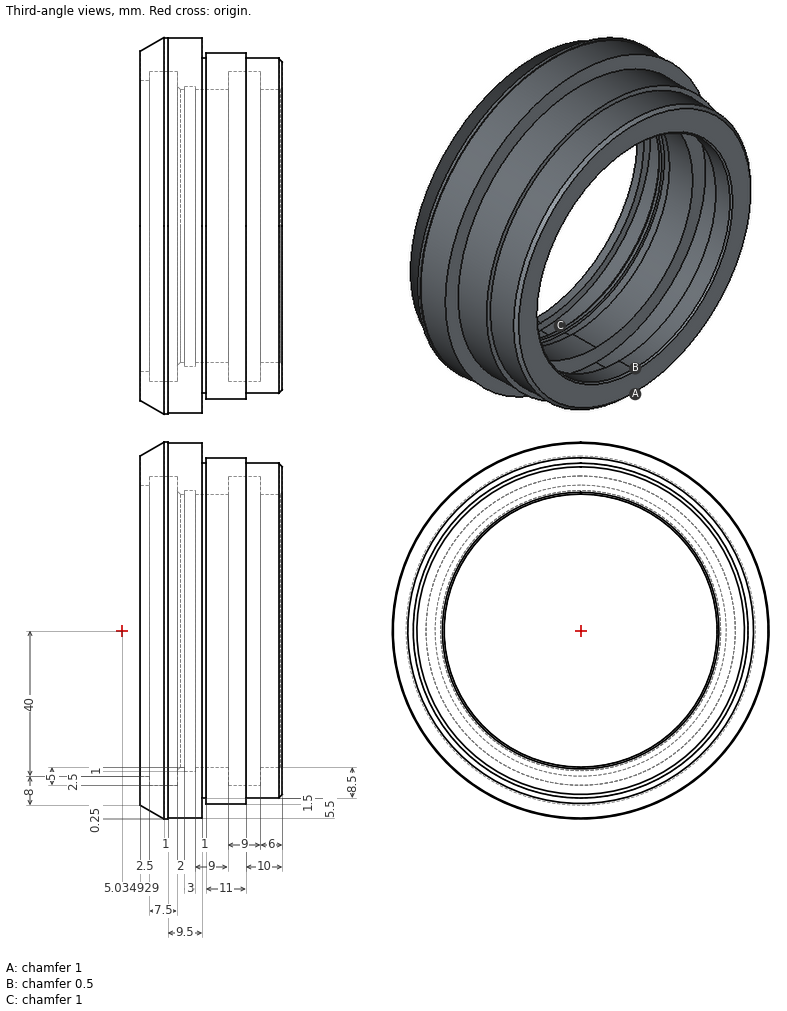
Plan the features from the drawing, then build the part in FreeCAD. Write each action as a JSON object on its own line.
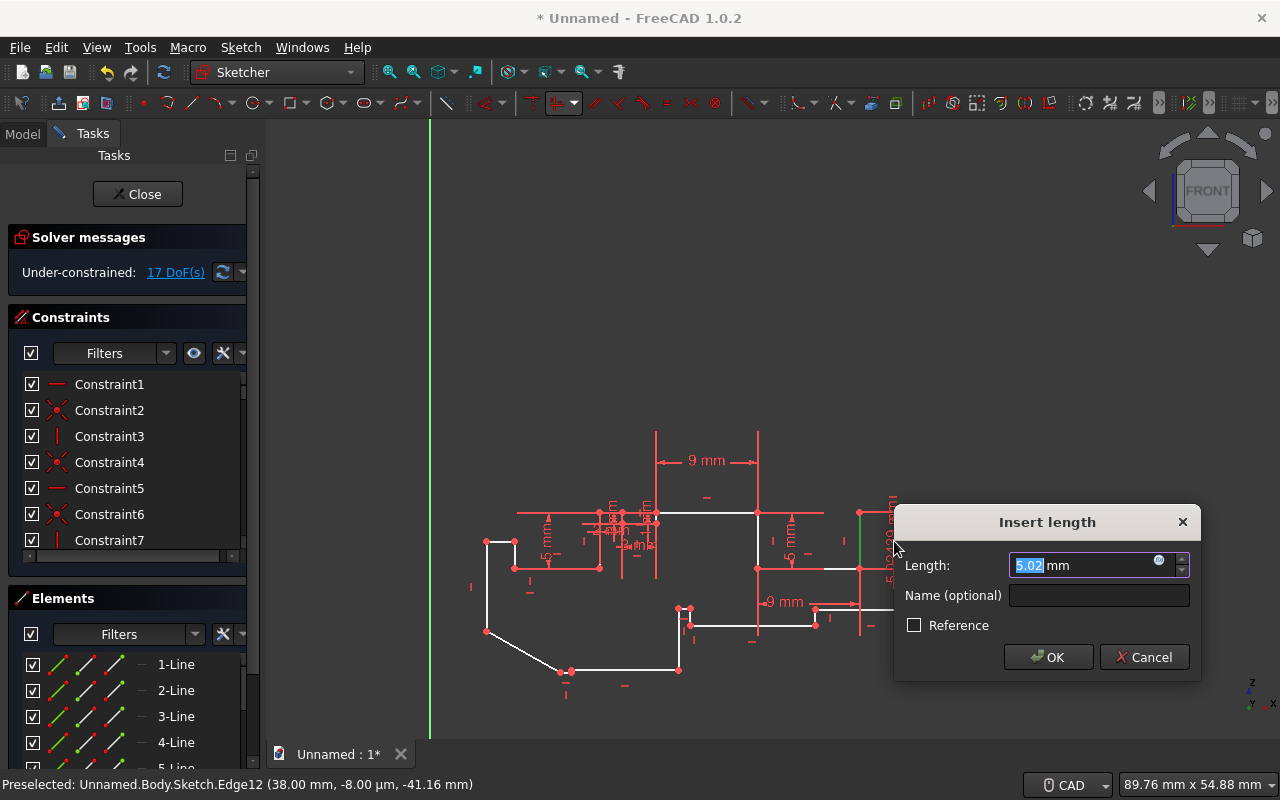
{"action": "type", "text": "5"}
{"action": "key", "text": "Return"}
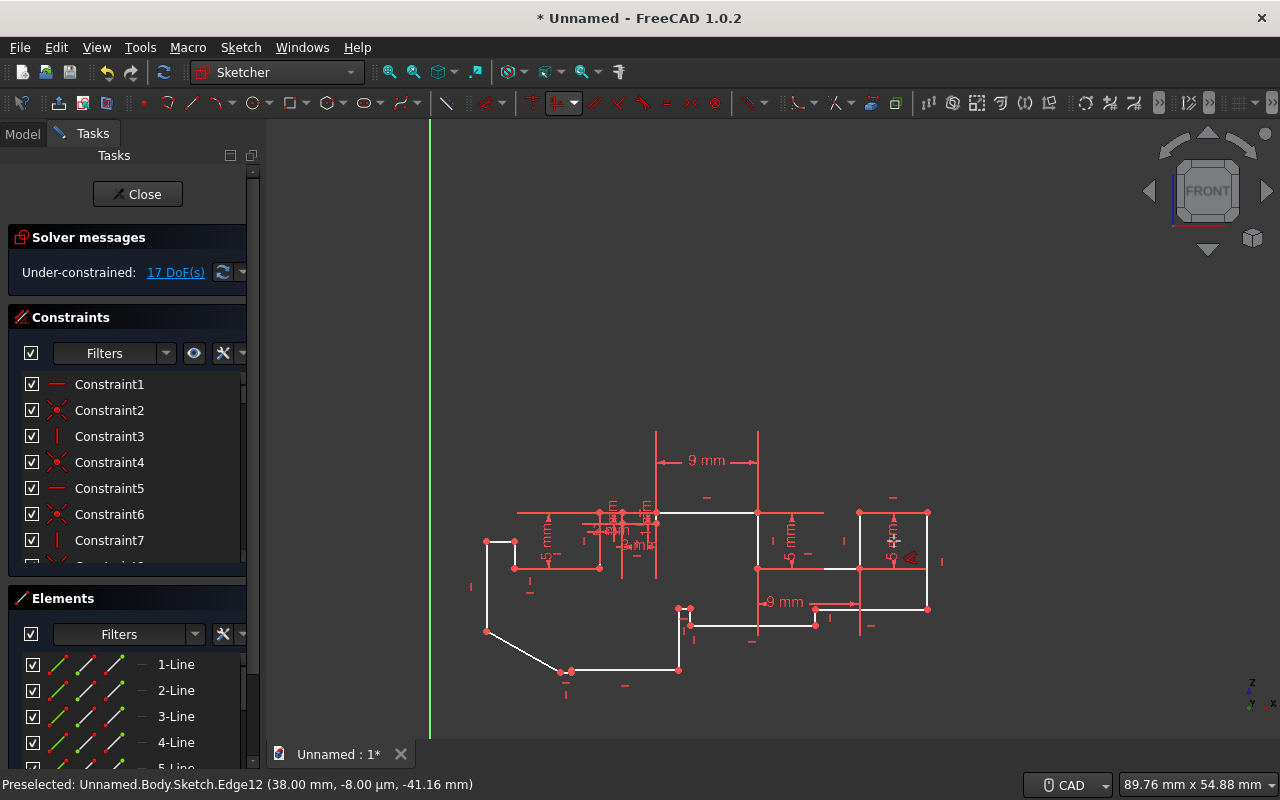
{"action": "left_click", "coordinate": [880, 513]}
{"action": "left_click", "coordinate": [893, 479]}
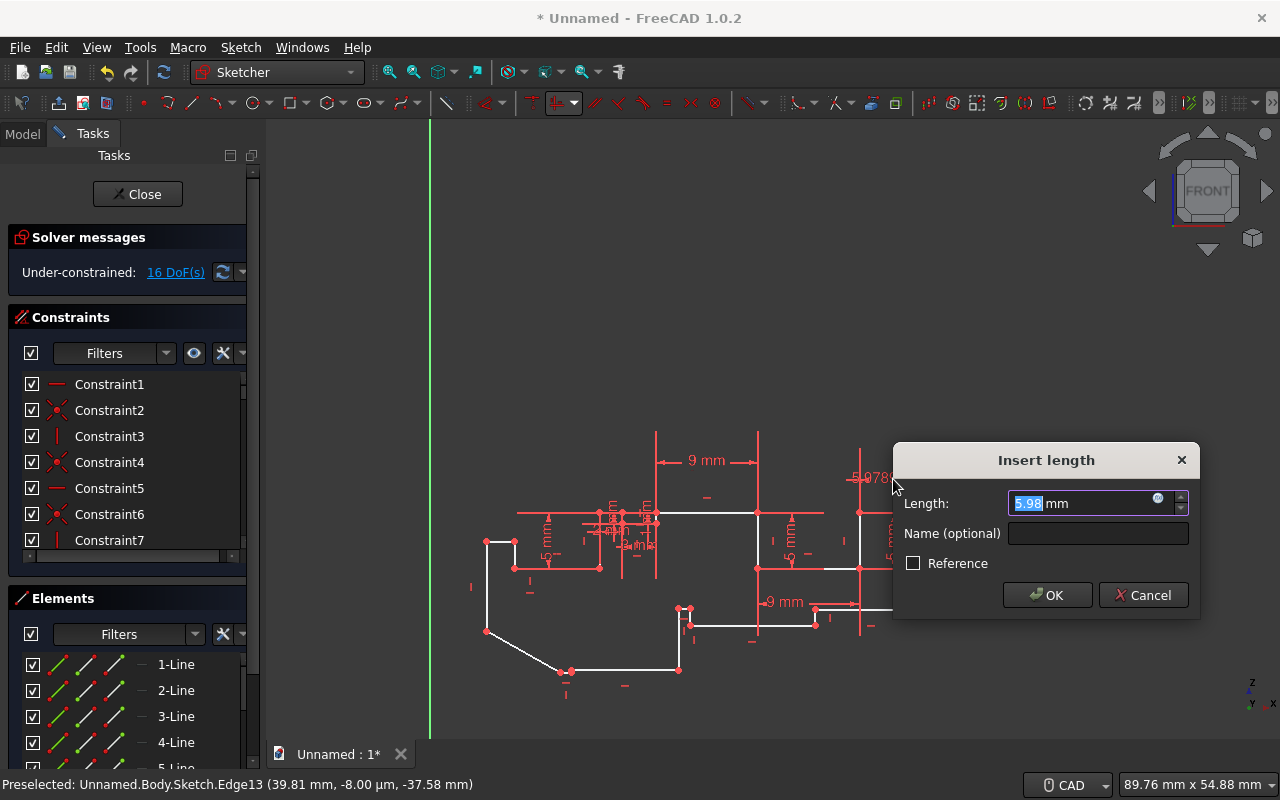
{"action": "type", "text": "6"}
{"action": "key", "text": "Return"}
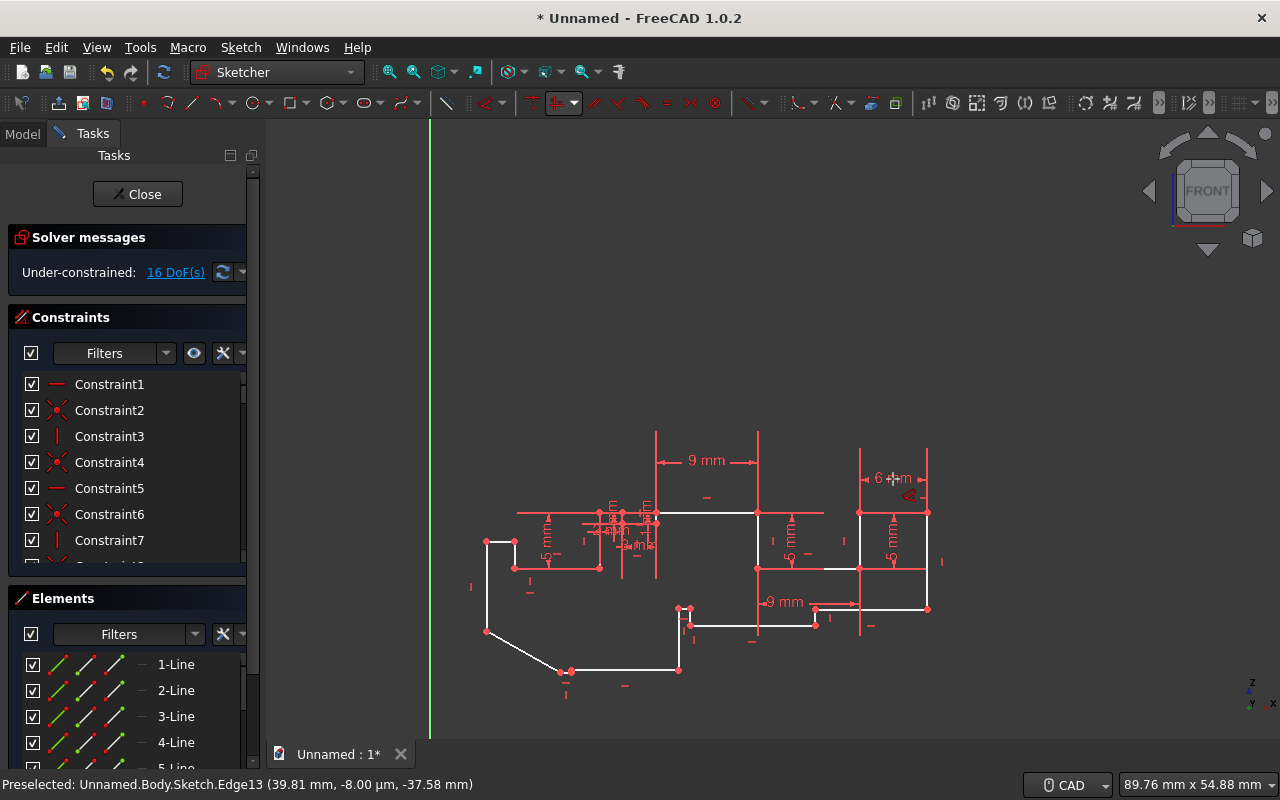
{"action": "scroll", "coordinate": [685, 609], "scroll_direction": "up", "scroll_amount": 7}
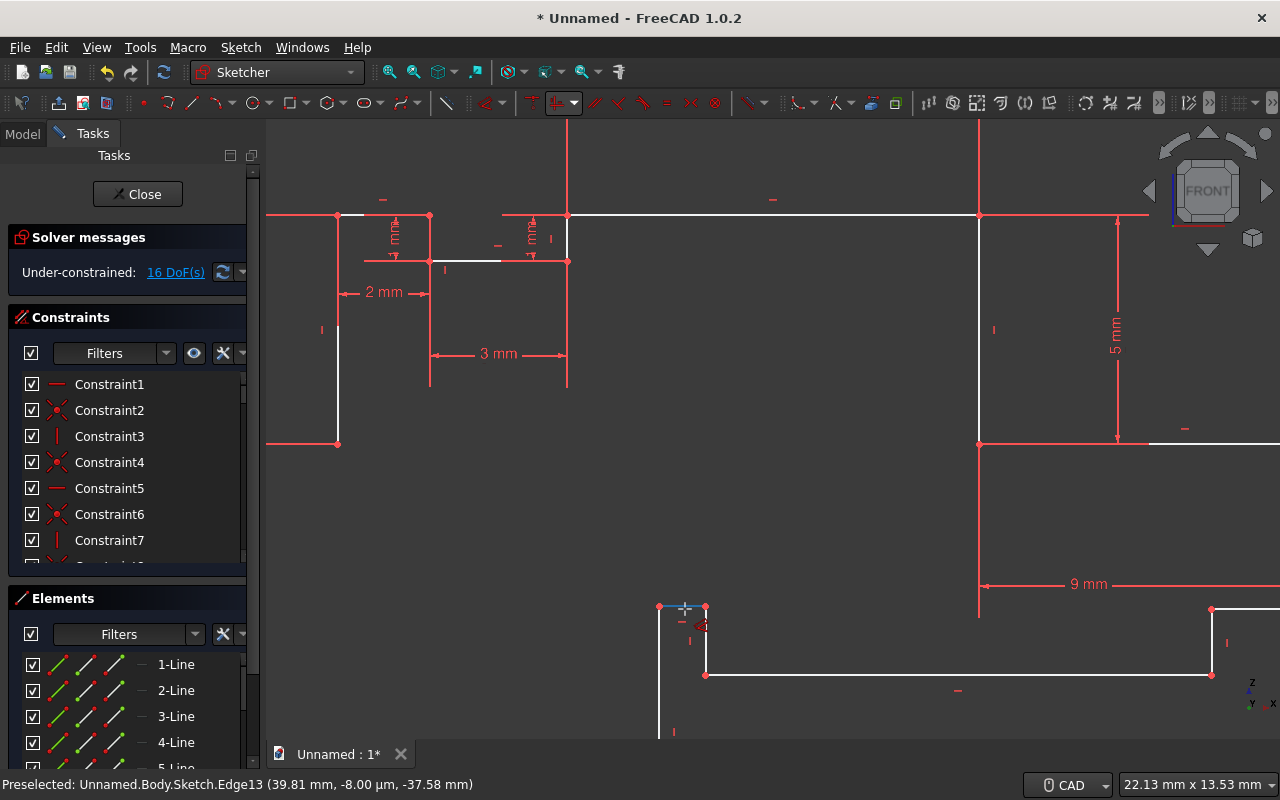
{"action": "left_click", "coordinate": [683, 606]}
{"action": "left_click", "coordinate": [683, 640]}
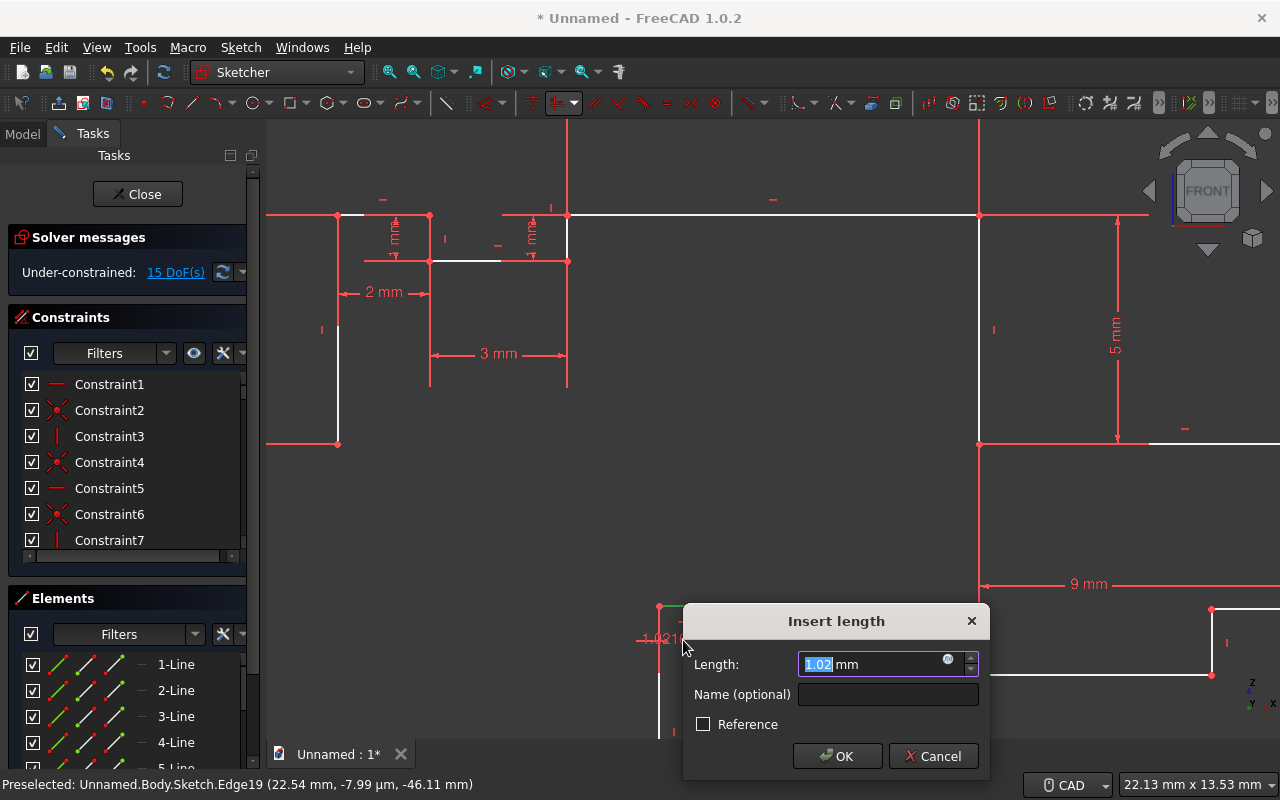
{"action": "type", "text": "1"}
{"action": "key", "text": "Return"}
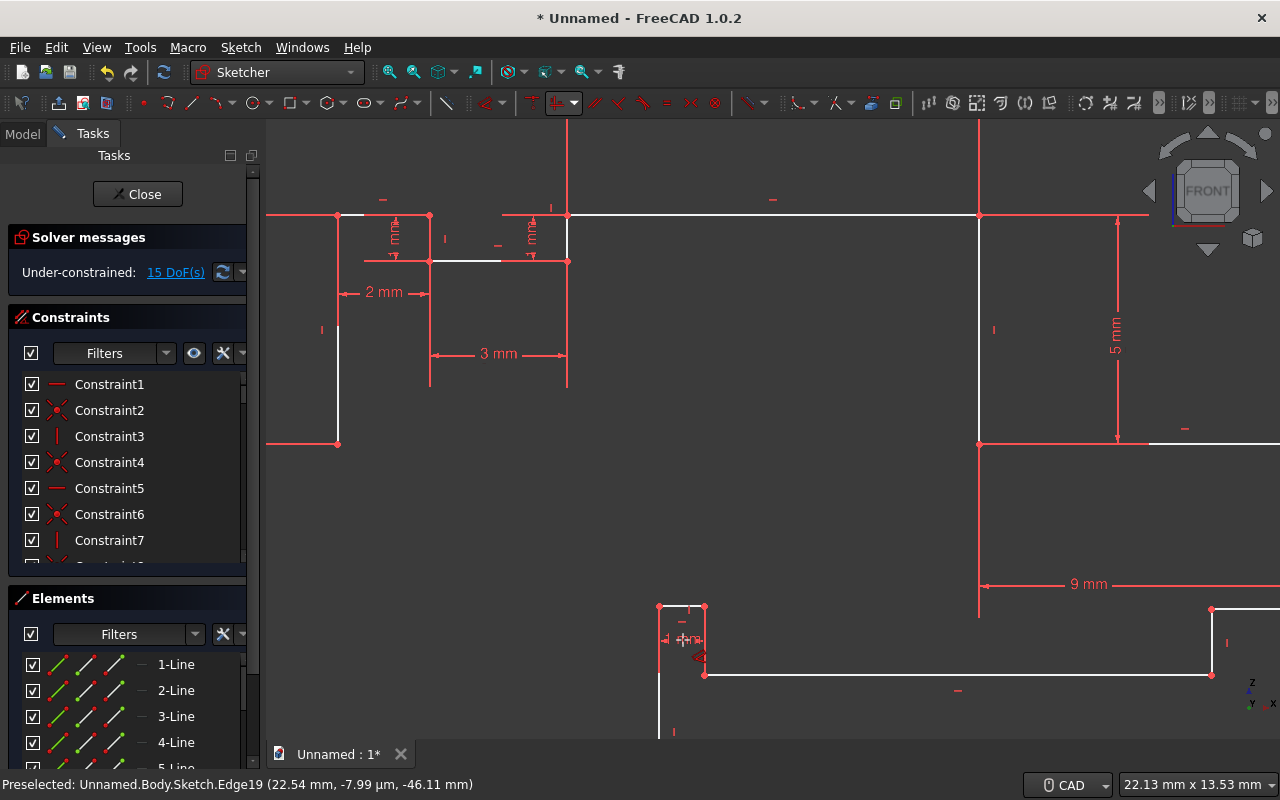
{"action": "scroll", "coordinate": [713, 577], "scroll_direction": "down", "scroll_amount": 9}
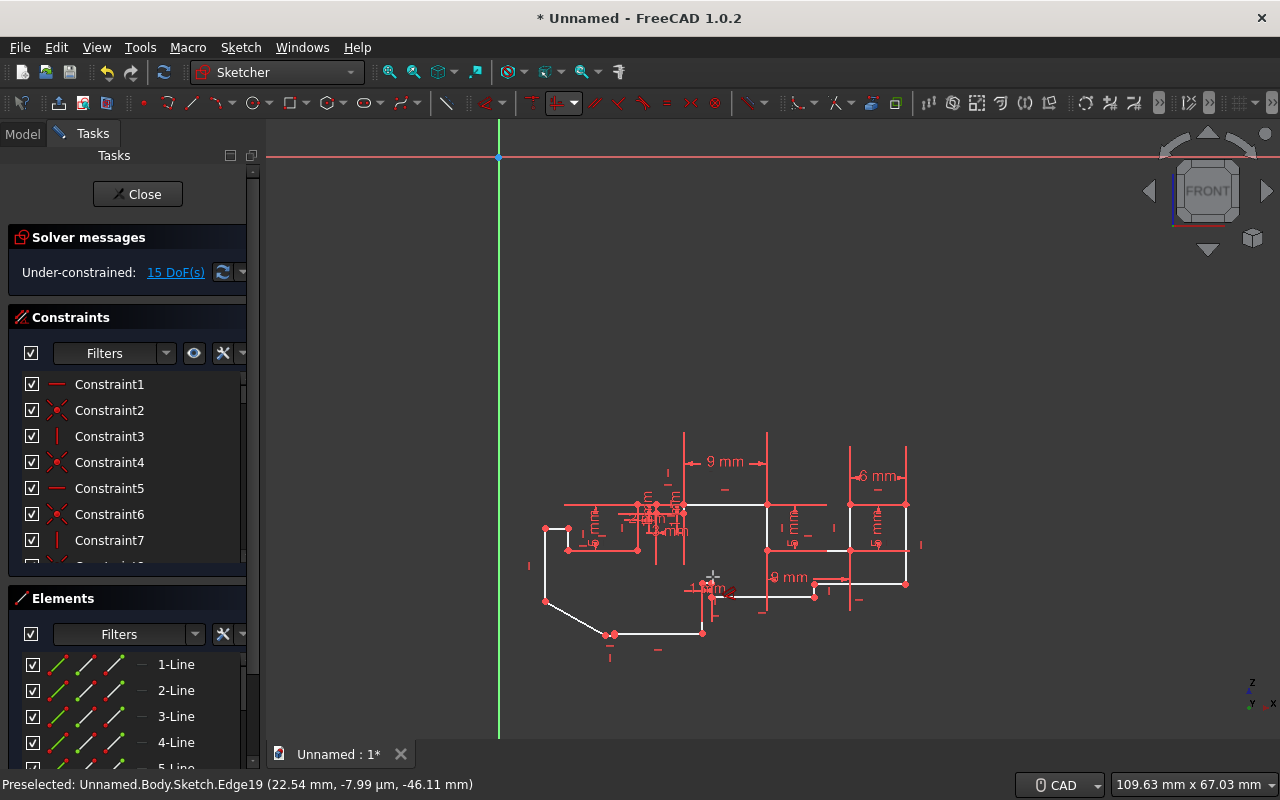
{"action": "scroll", "coordinate": [630, 625], "scroll_direction": "up", "scroll_amount": 10}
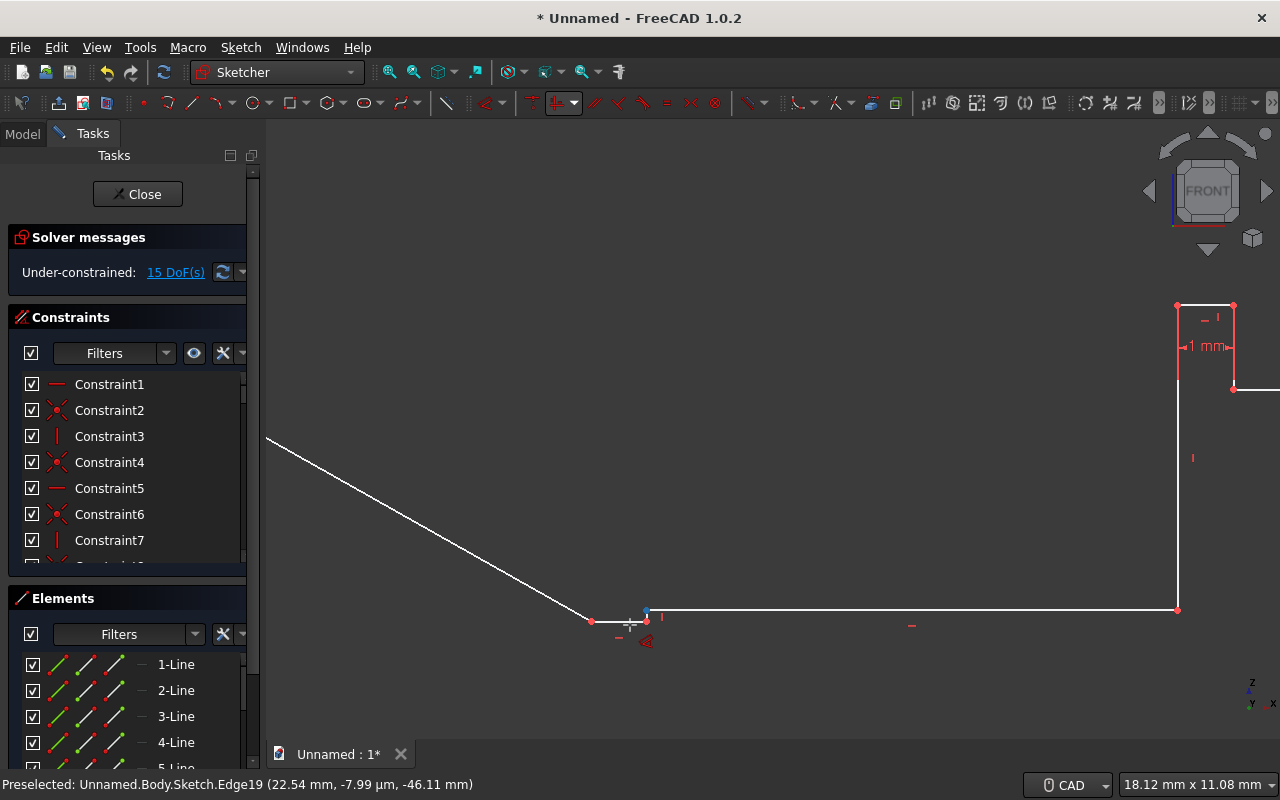
{"action": "left_click", "coordinate": [630, 622]}
{"action": "left_click", "coordinate": [619, 656]}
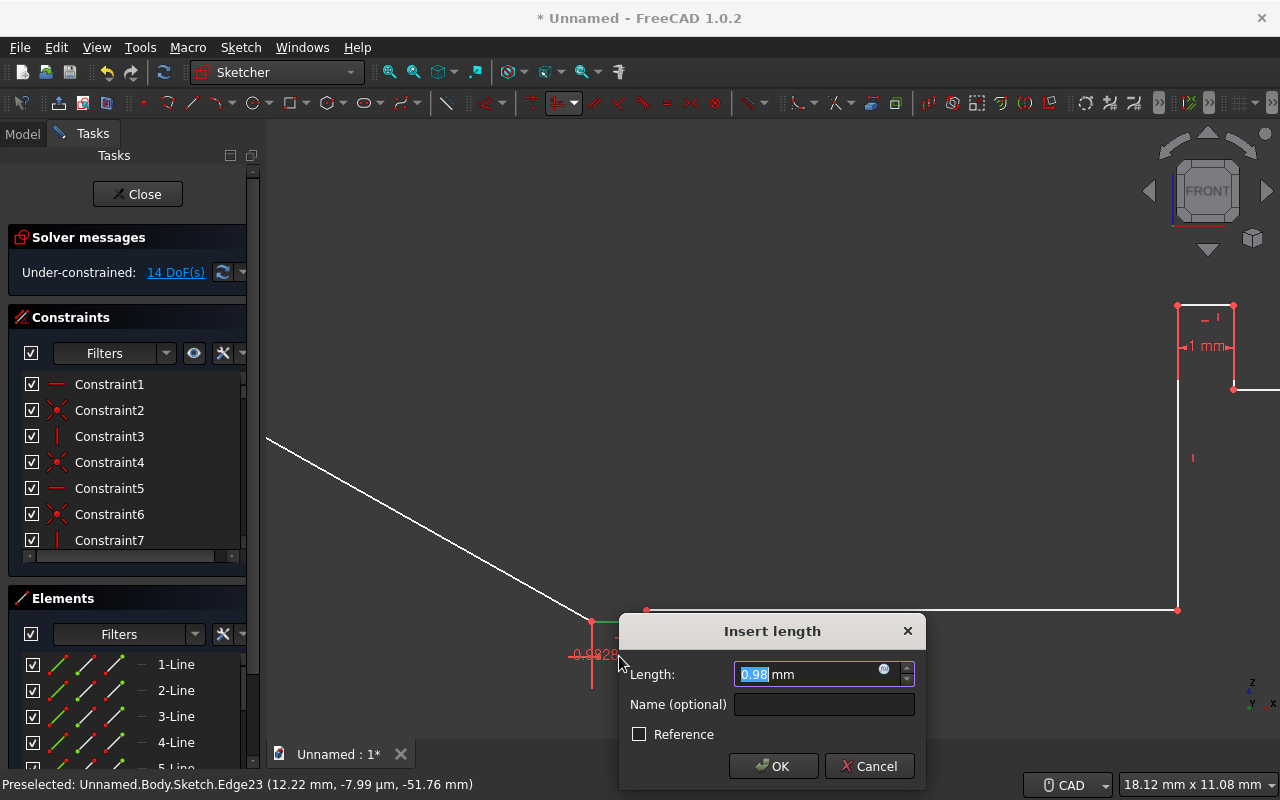
{"action": "type", "text": "1"}
{"action": "key", "text": "Return"}